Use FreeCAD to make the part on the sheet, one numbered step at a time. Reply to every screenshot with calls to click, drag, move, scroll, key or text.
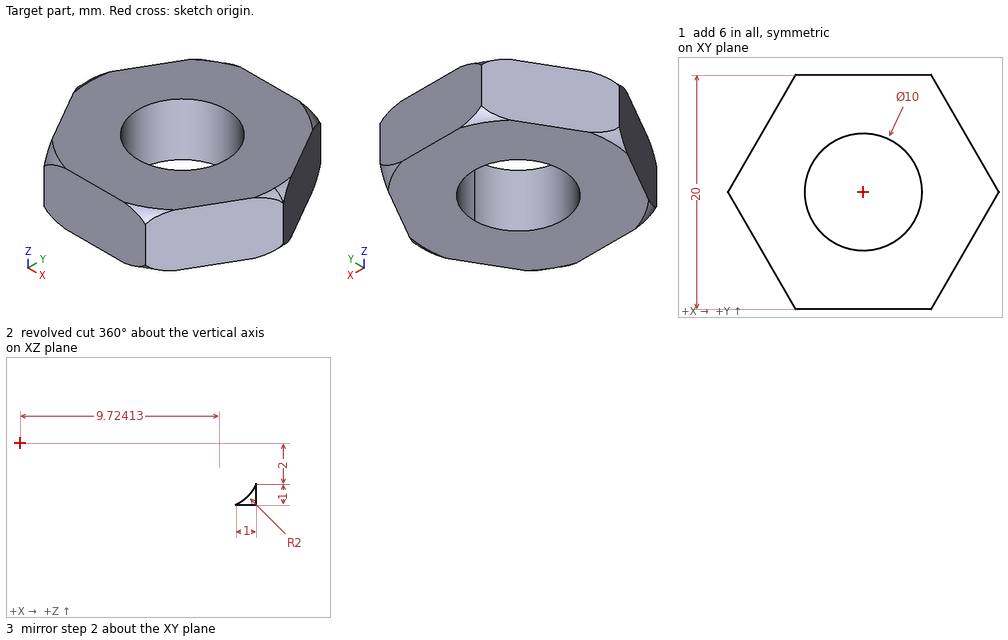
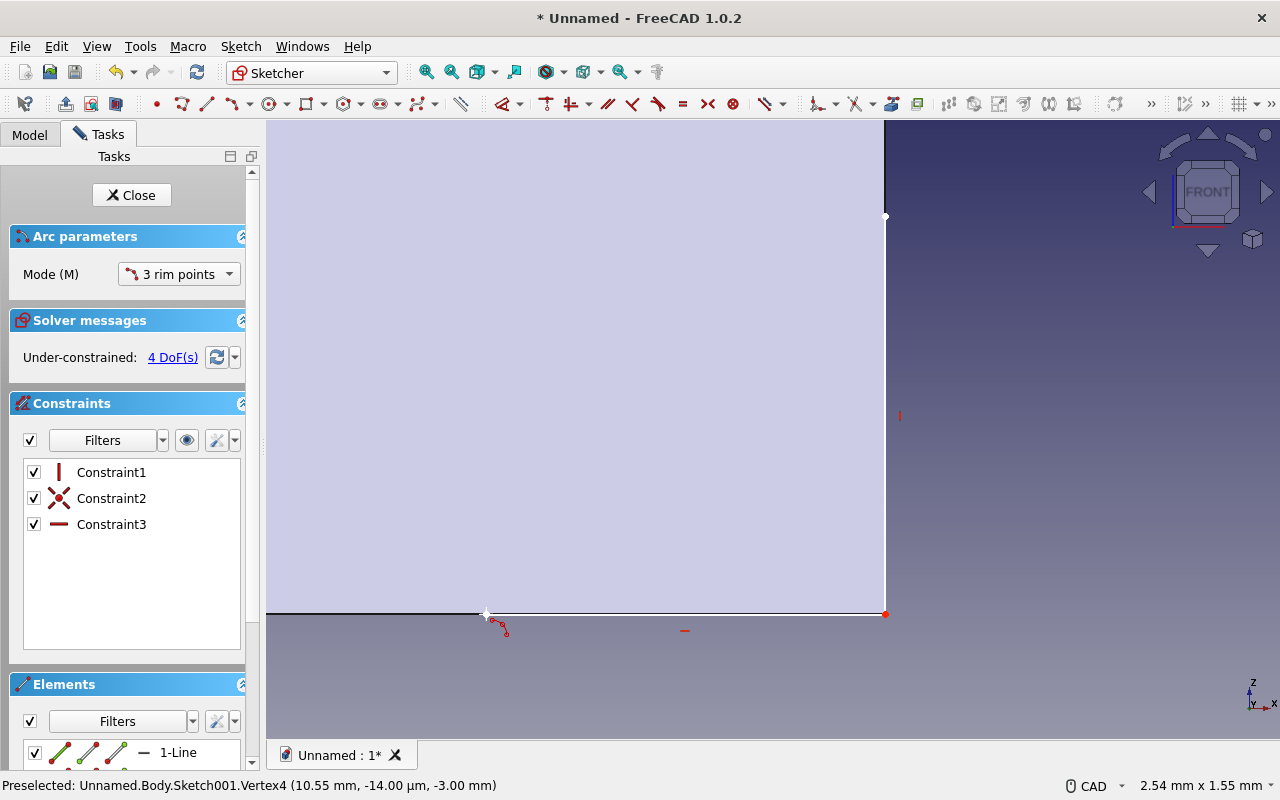
click(486, 615)
click(885, 216)
click(722, 451)
key(Escape)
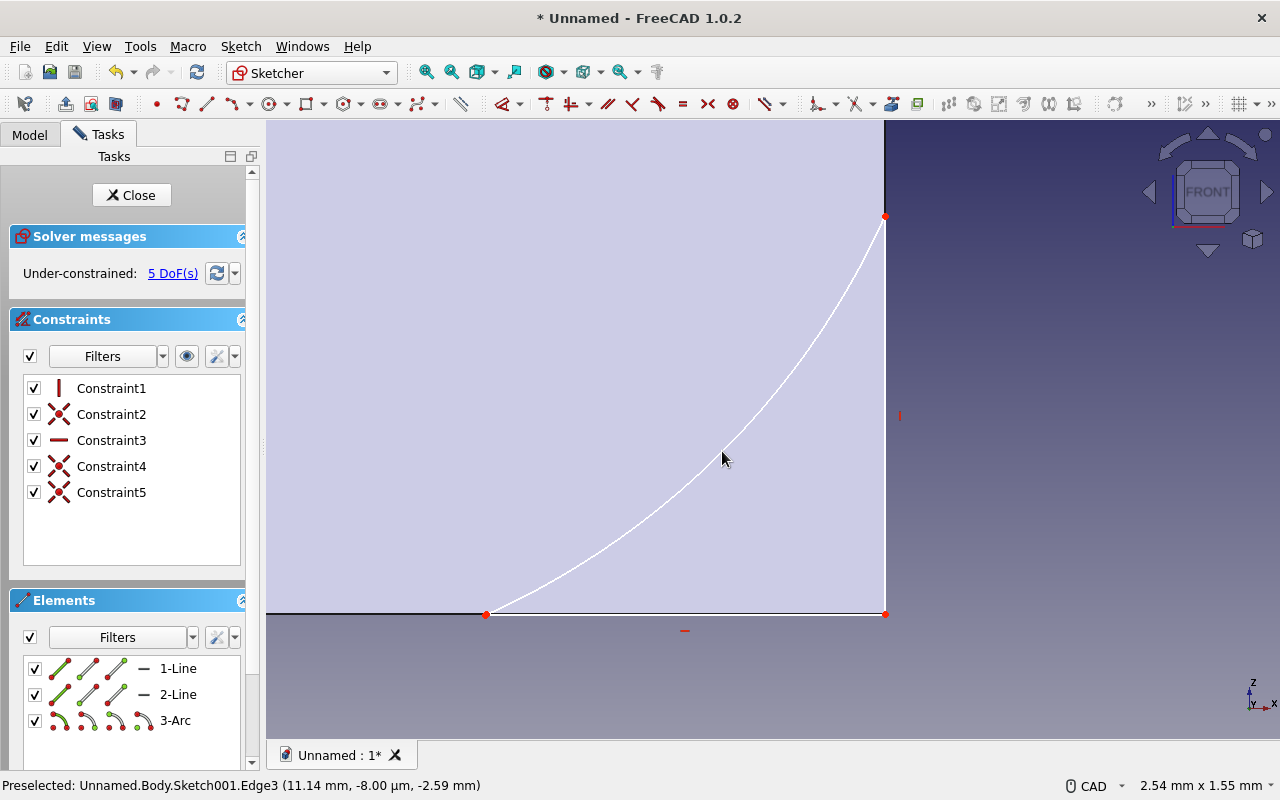
key(d)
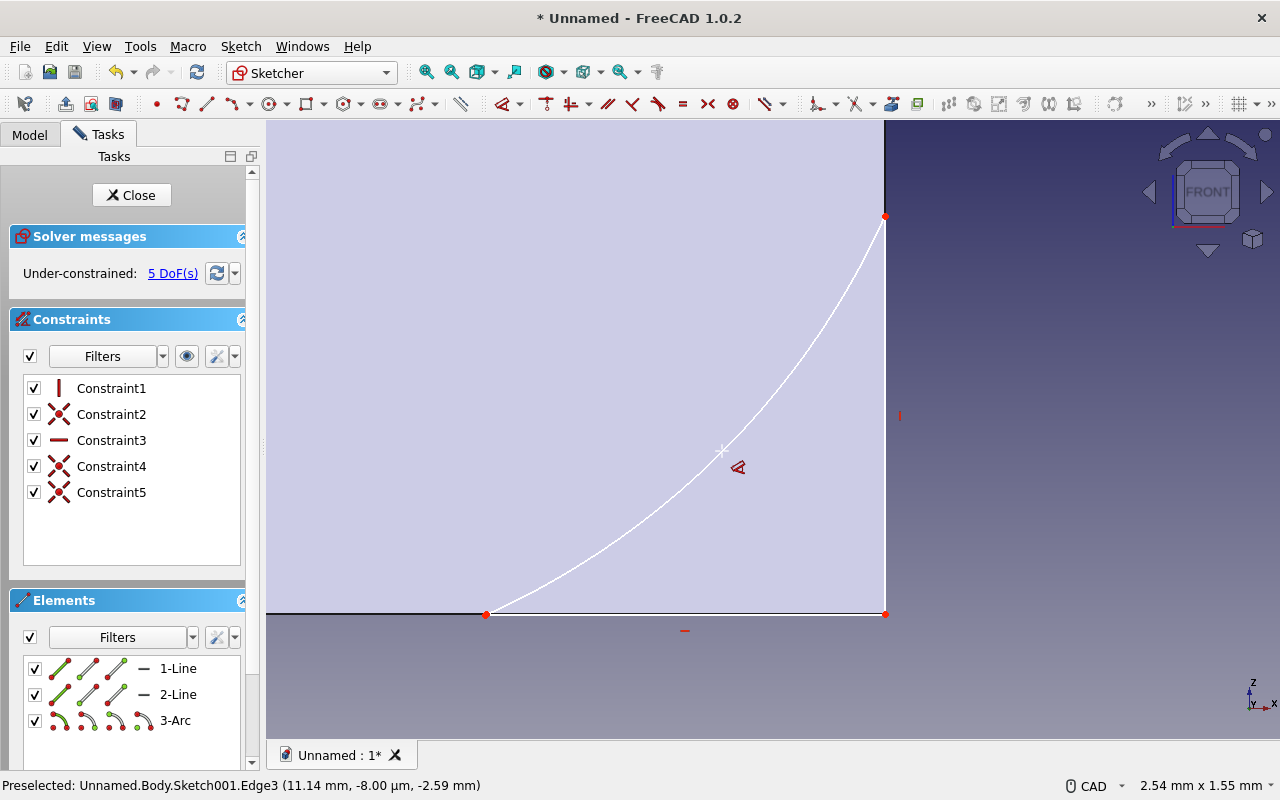
click(635, 527)
click(654, 553)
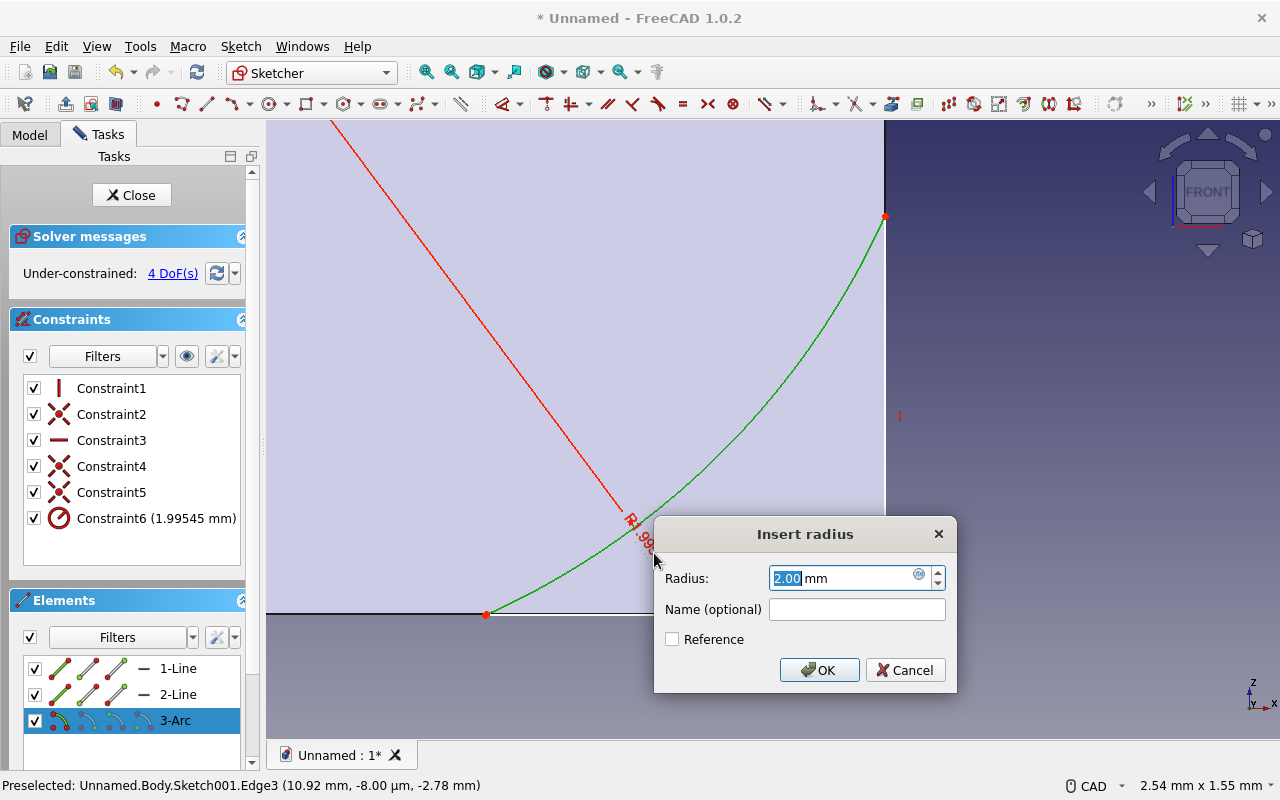
text(2)
key(Return)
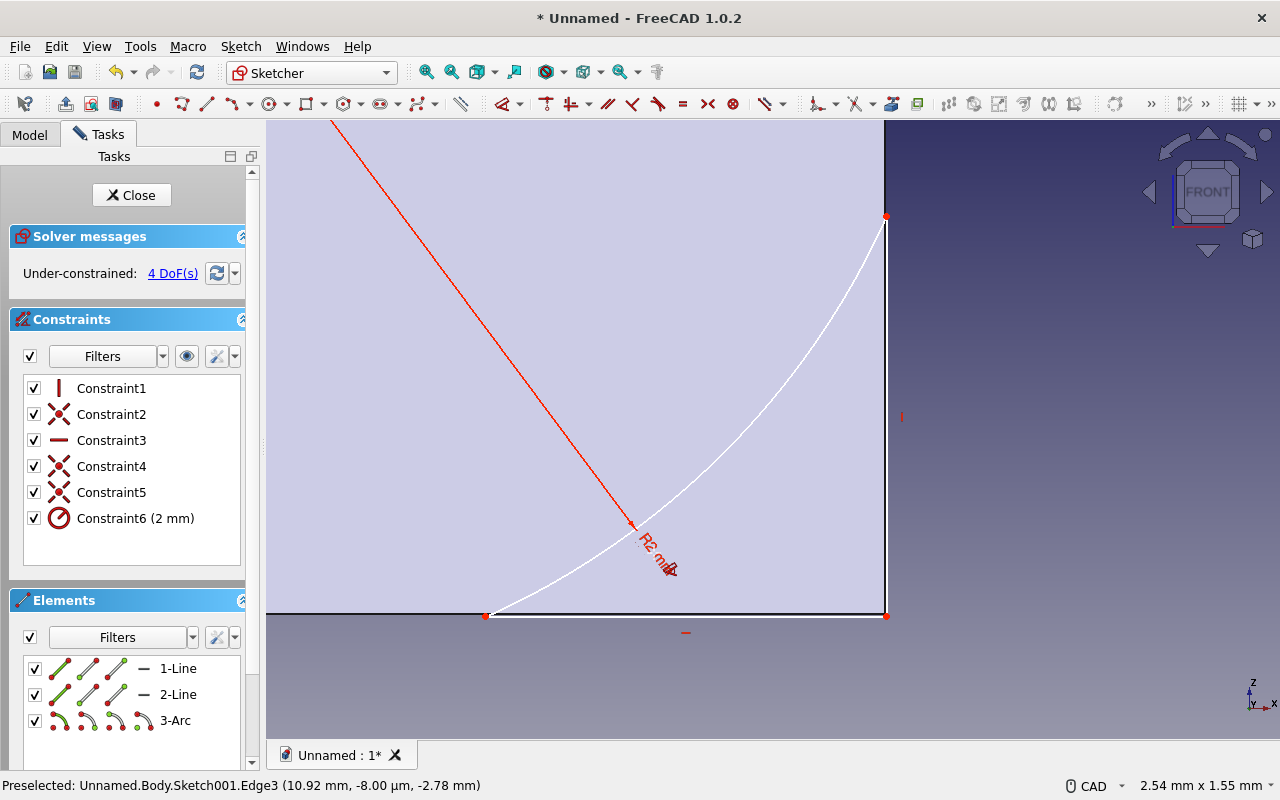
click(887, 336)
click(921, 416)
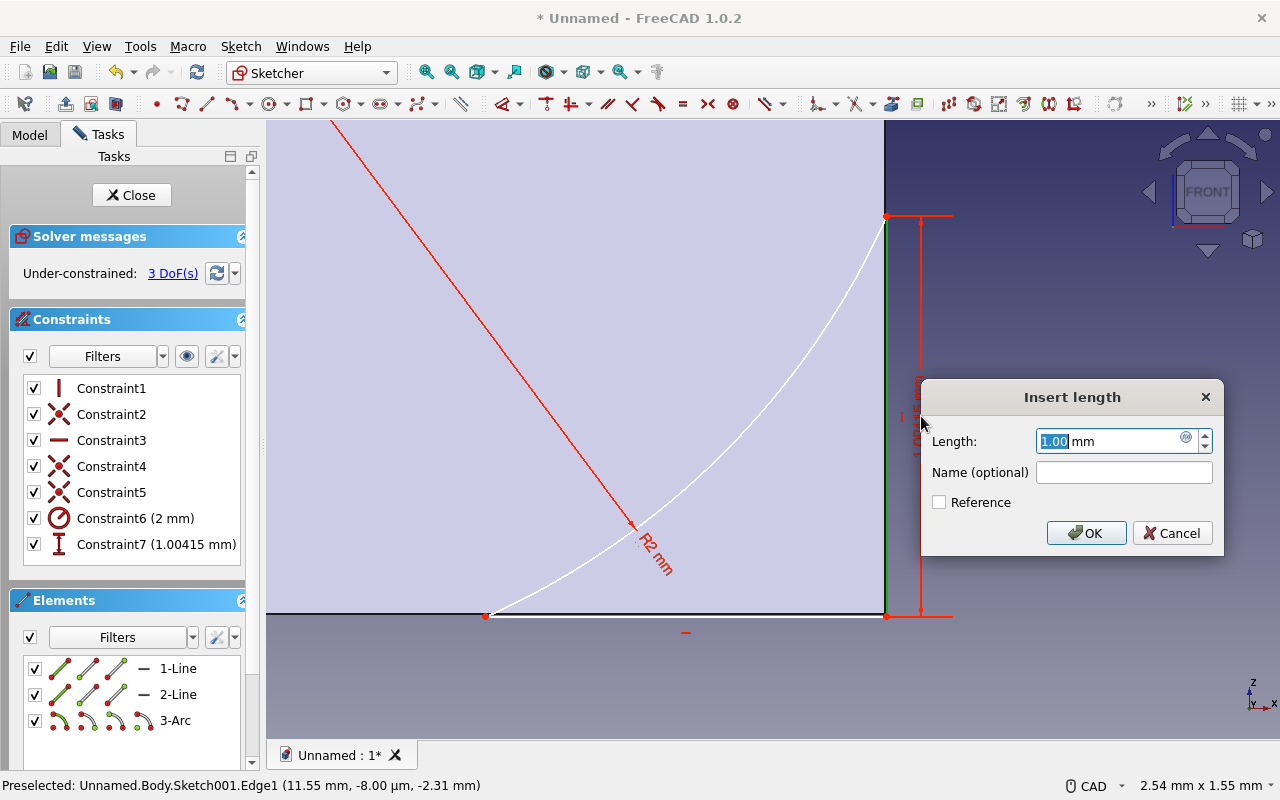
text(1)
key(Return)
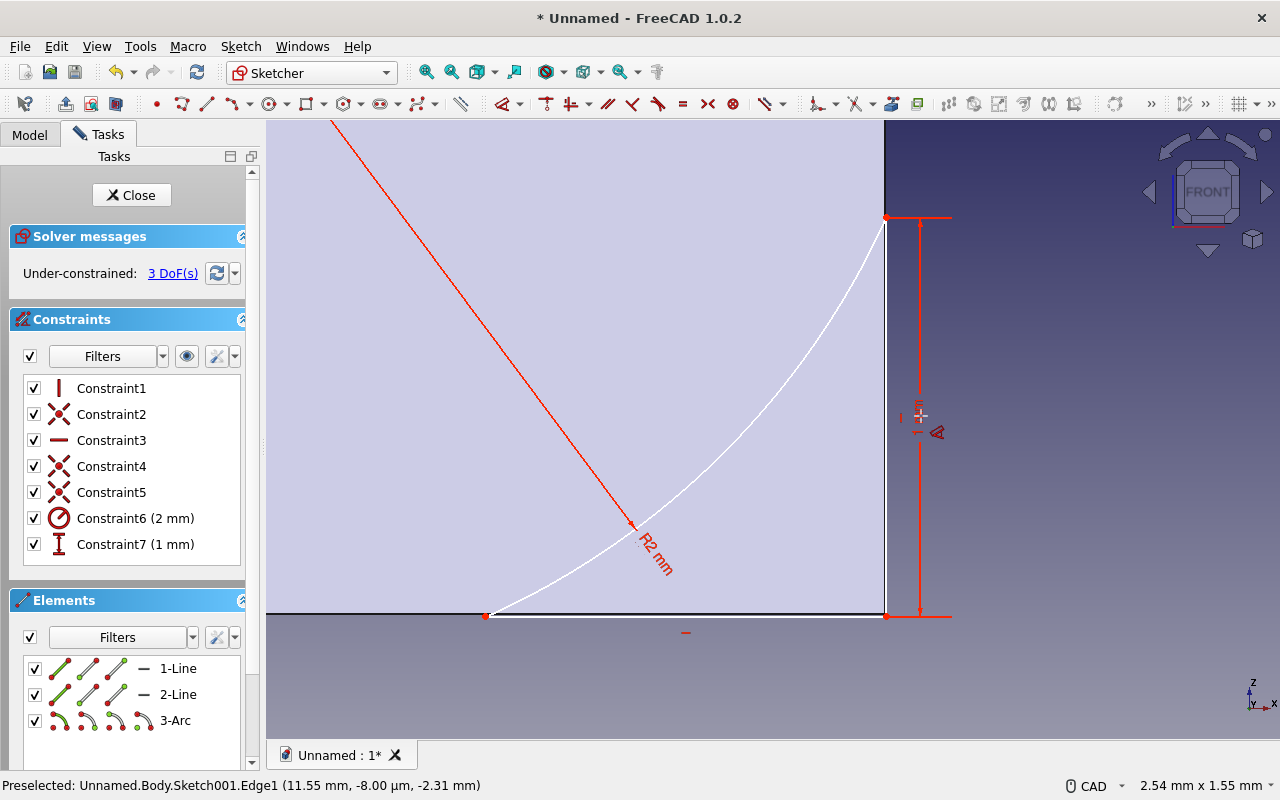
click(766, 617)
click(686, 651)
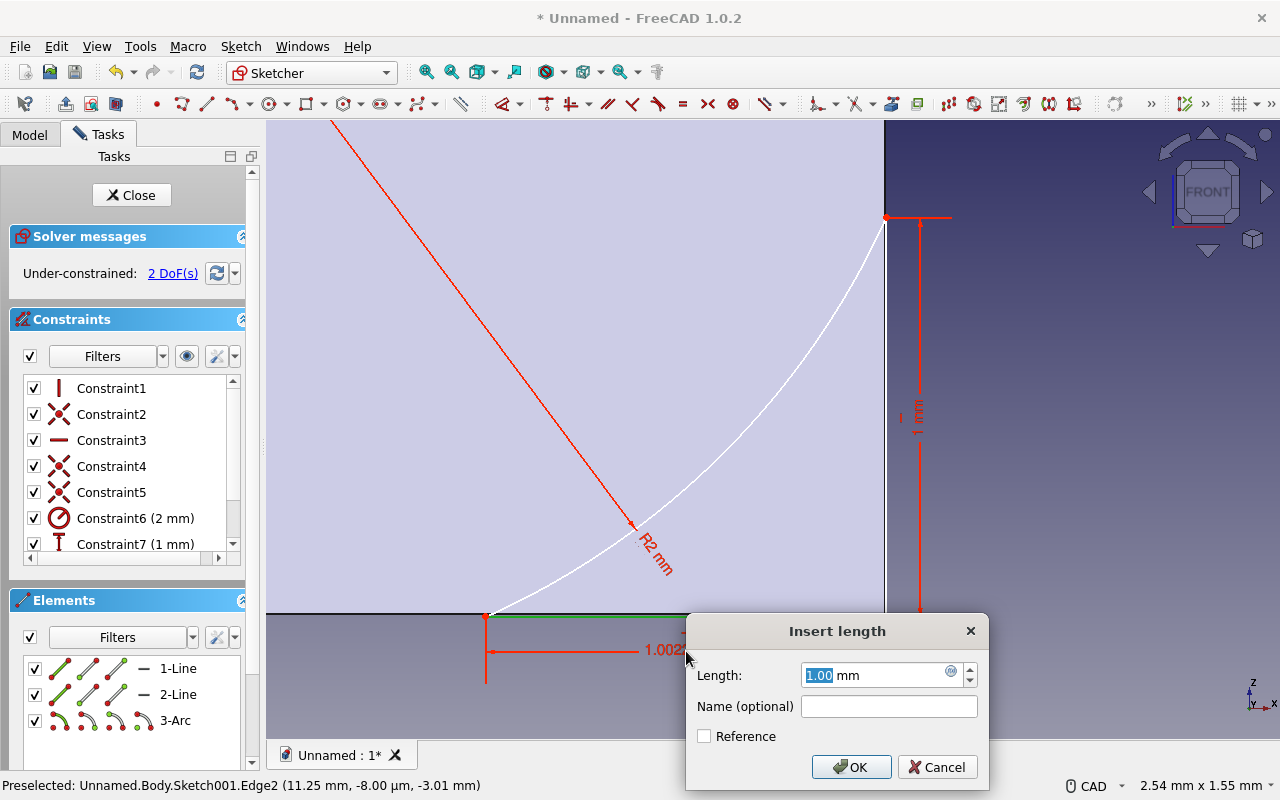
text(1)
key(Return)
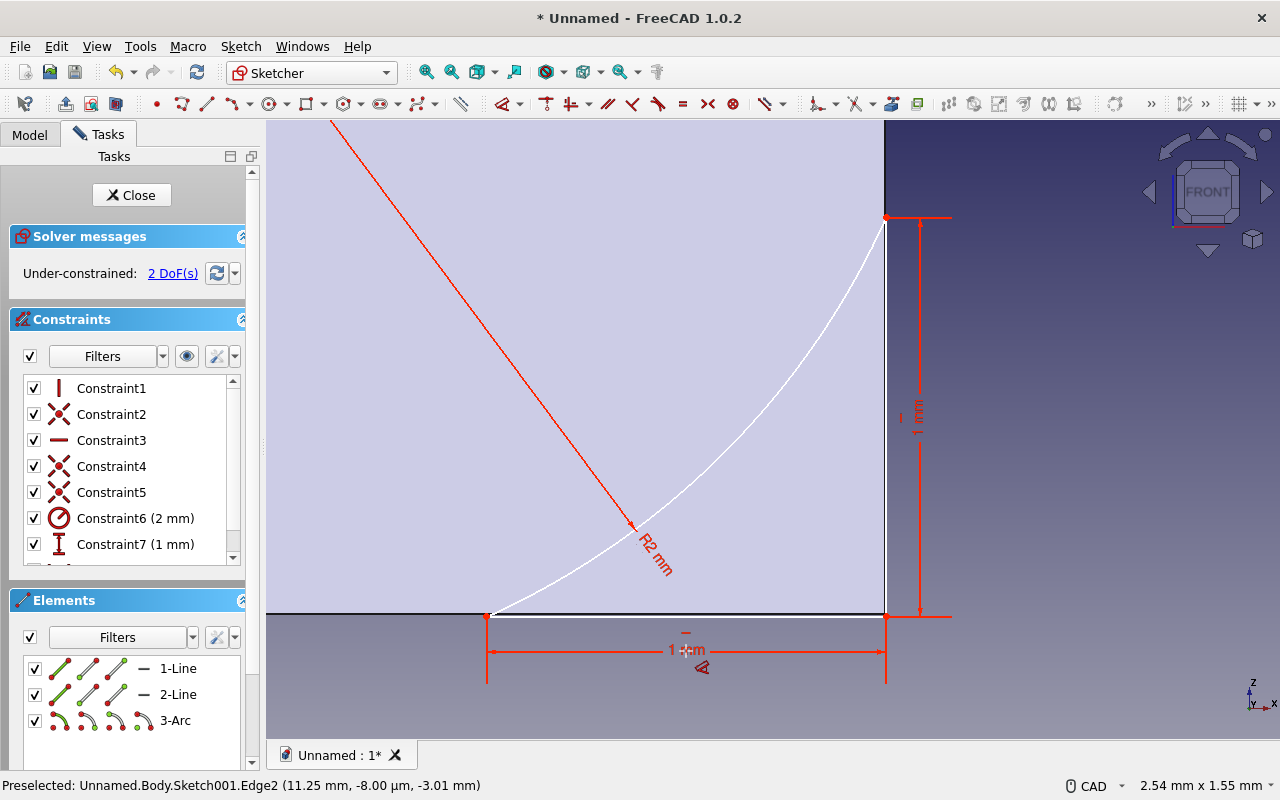
click(886, 218)
click(920, 183)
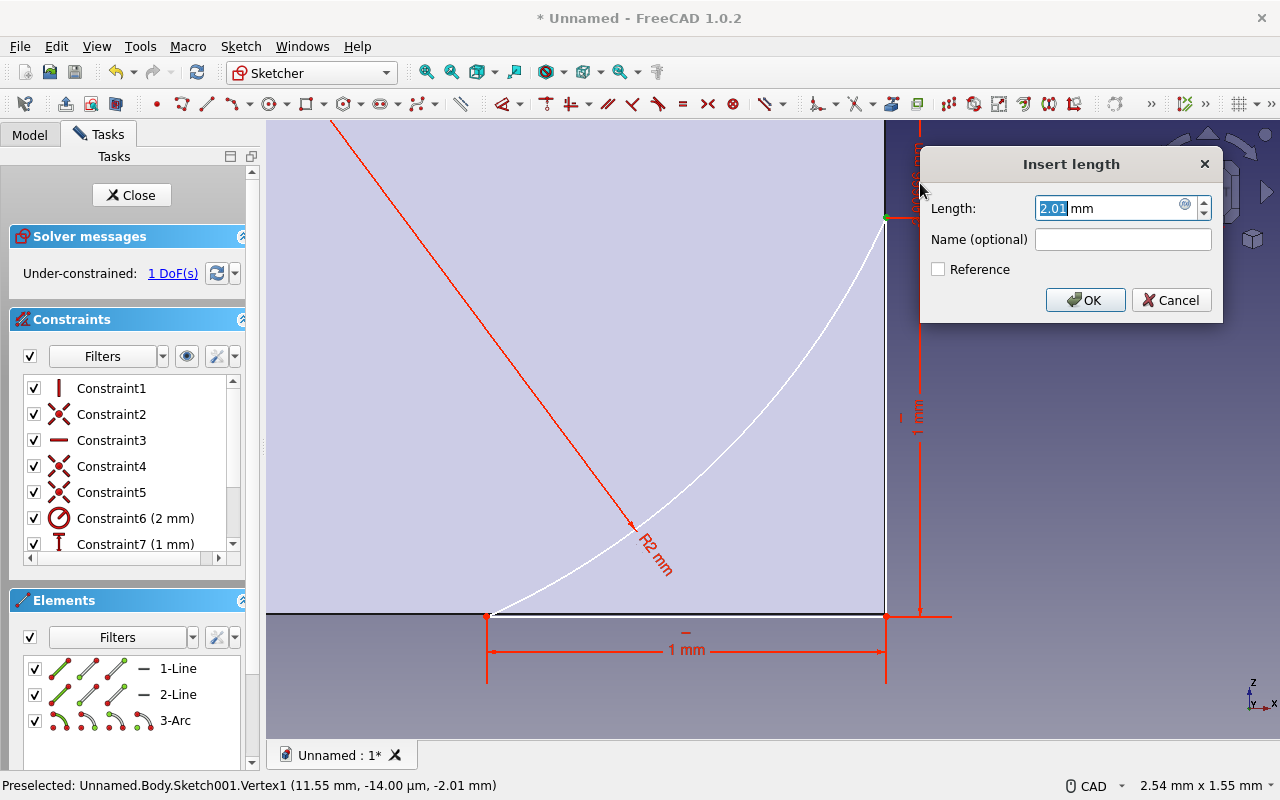
text(2)
key(Return)